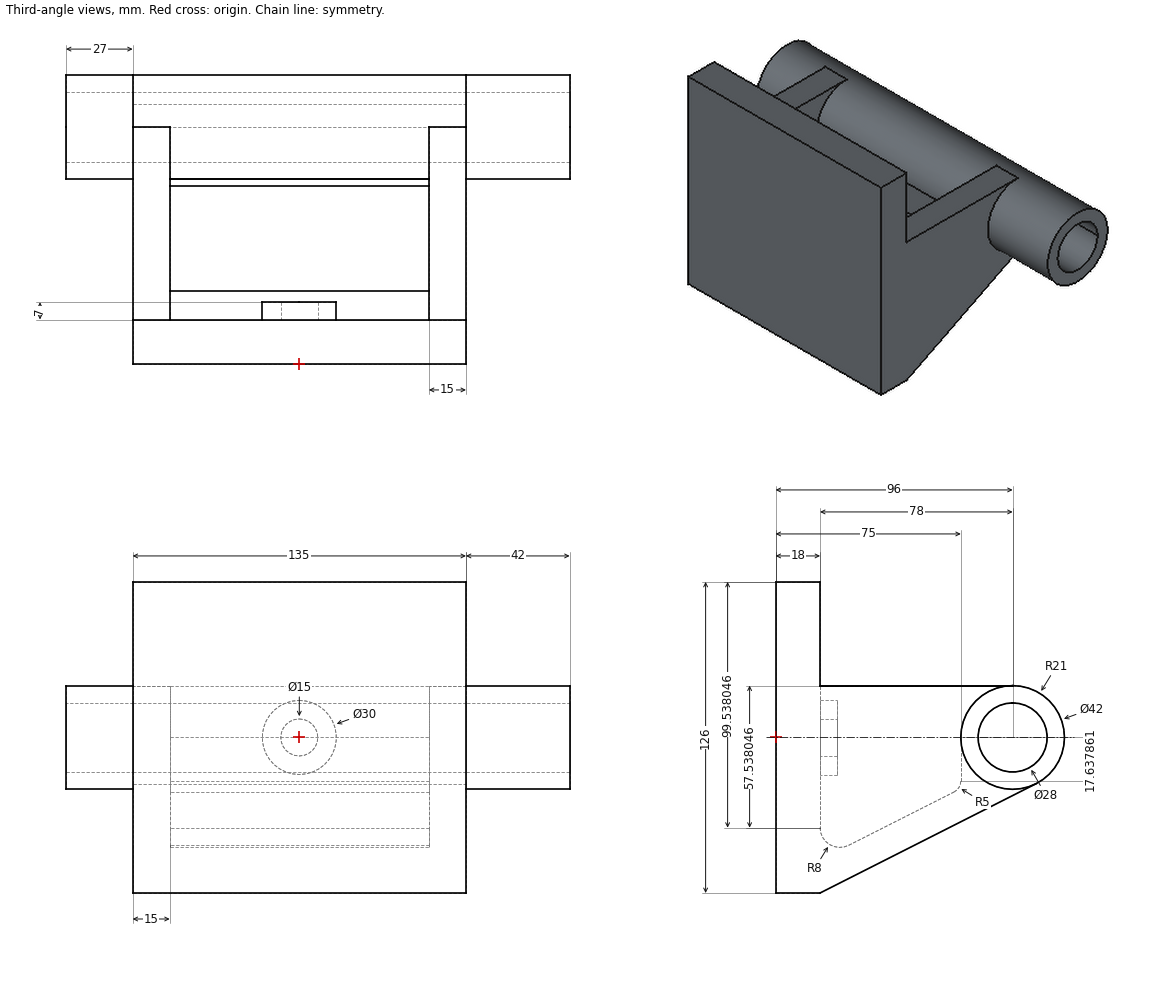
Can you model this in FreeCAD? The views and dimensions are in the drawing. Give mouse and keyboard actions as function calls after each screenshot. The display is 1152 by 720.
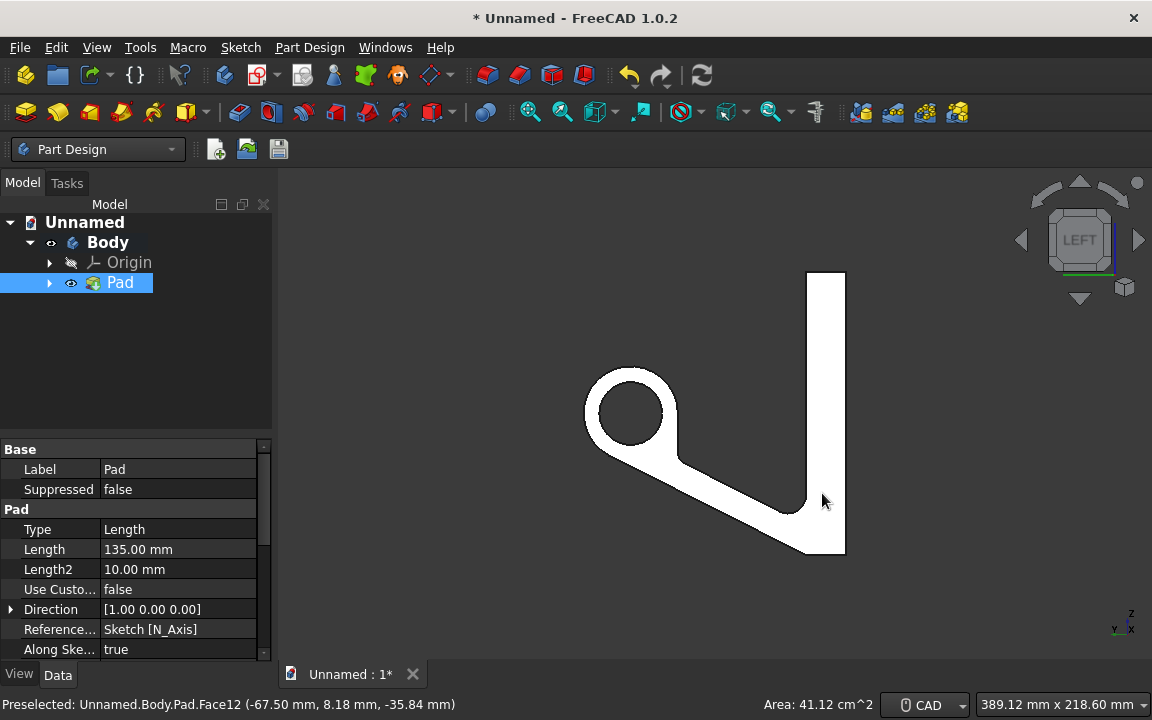
click(258, 76)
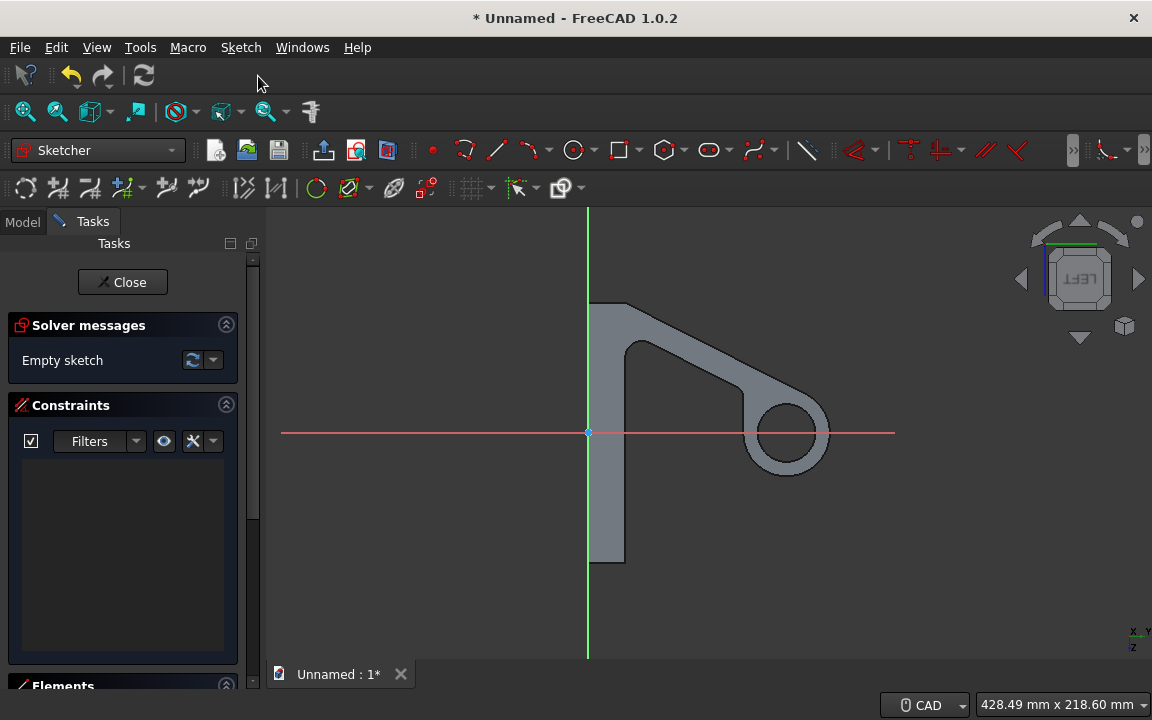
scroll(850, 433, up, 6)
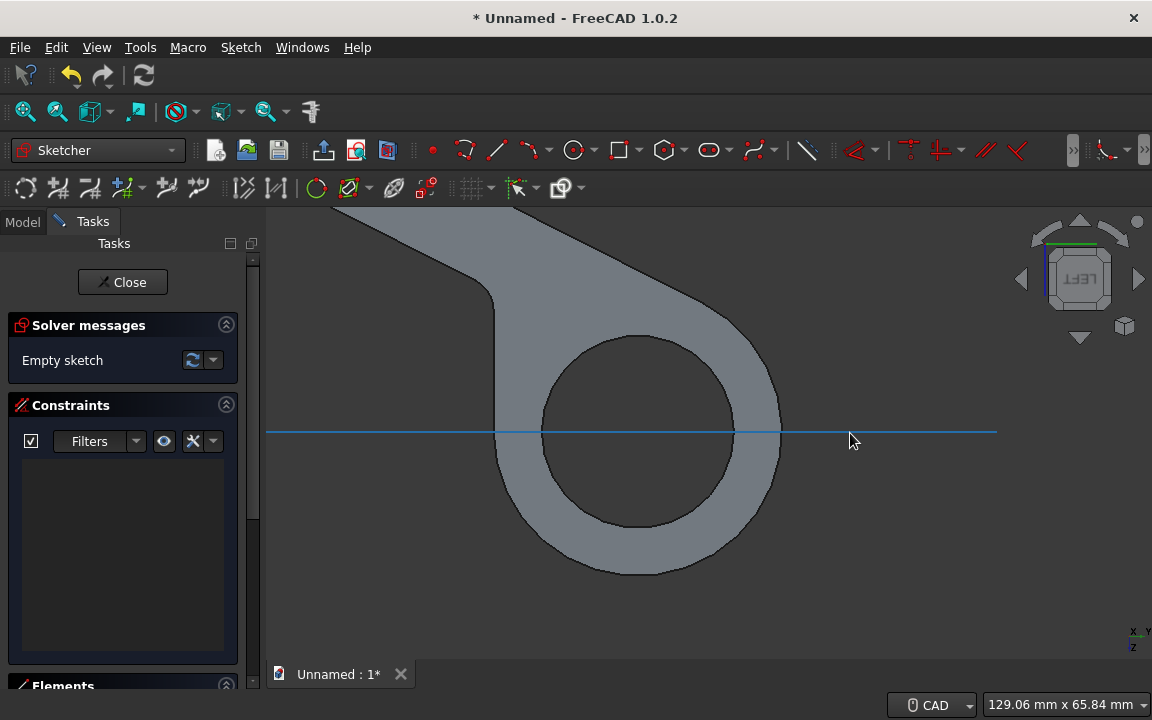
click(574, 150)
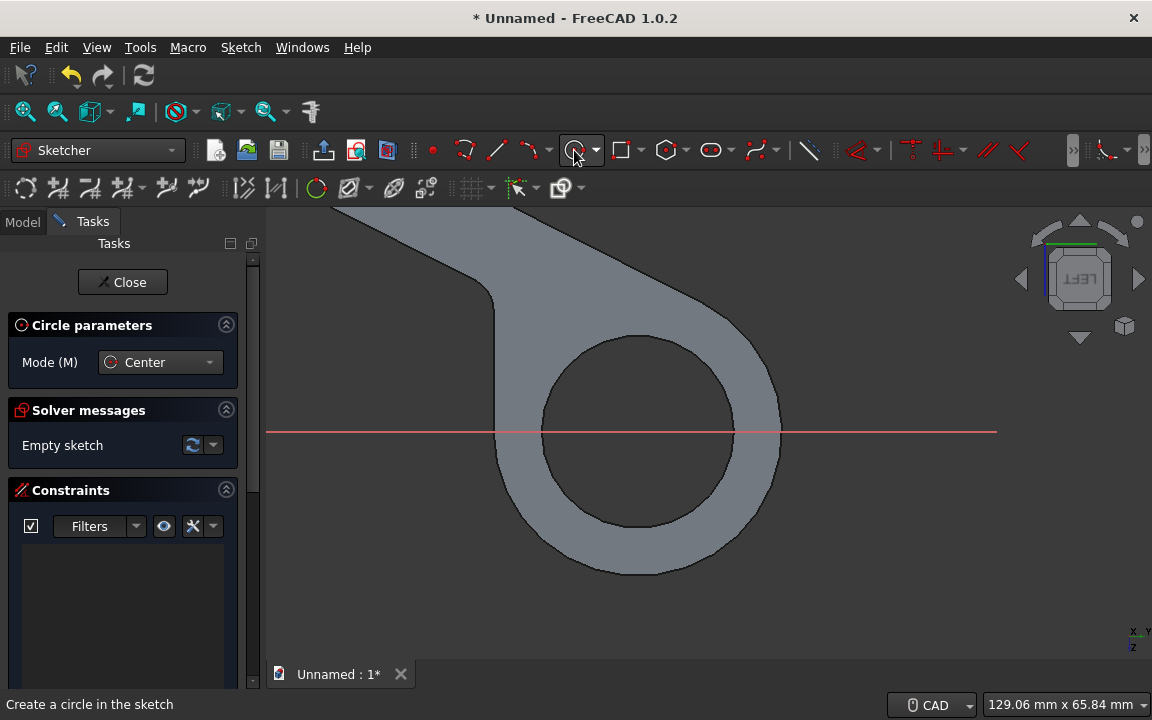
click(638, 432)
click(740, 330)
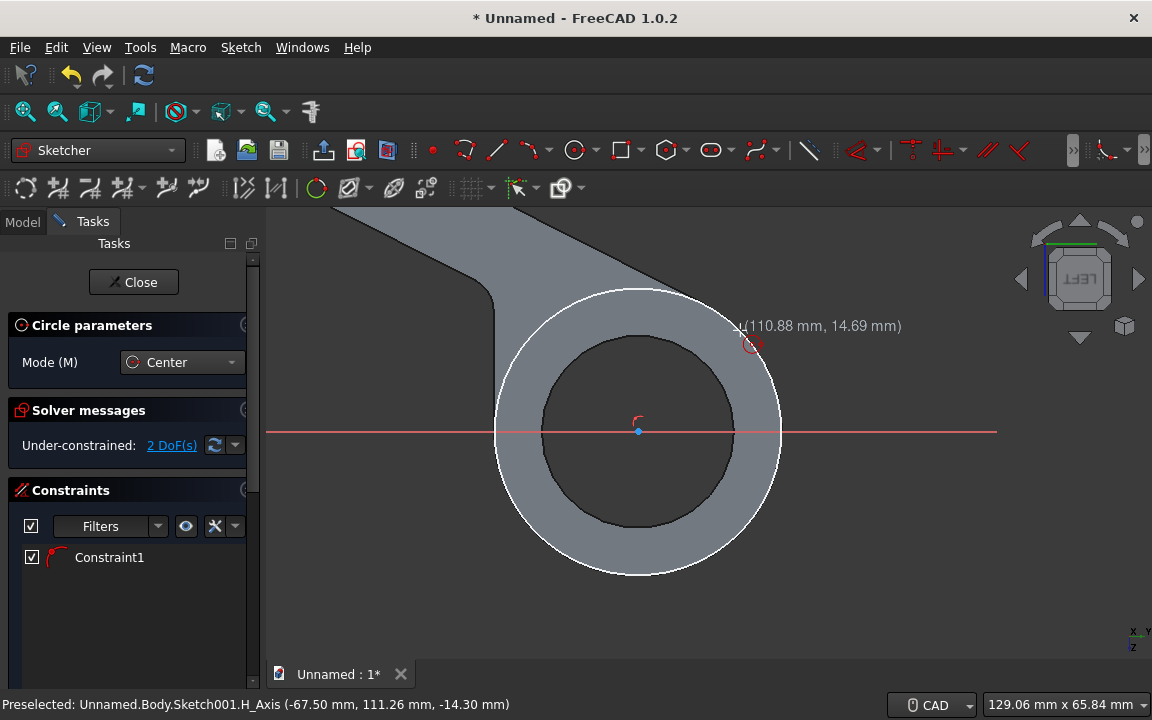
click(638, 432)
click(706, 364)
key(Escape)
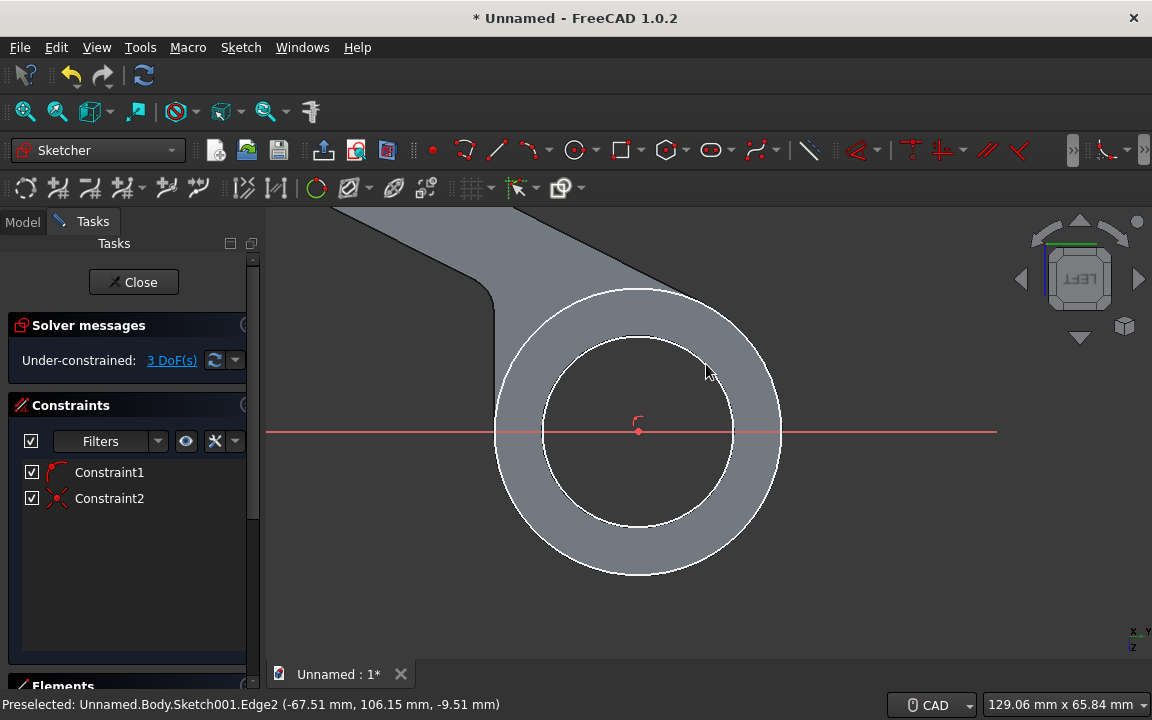
click(856, 150)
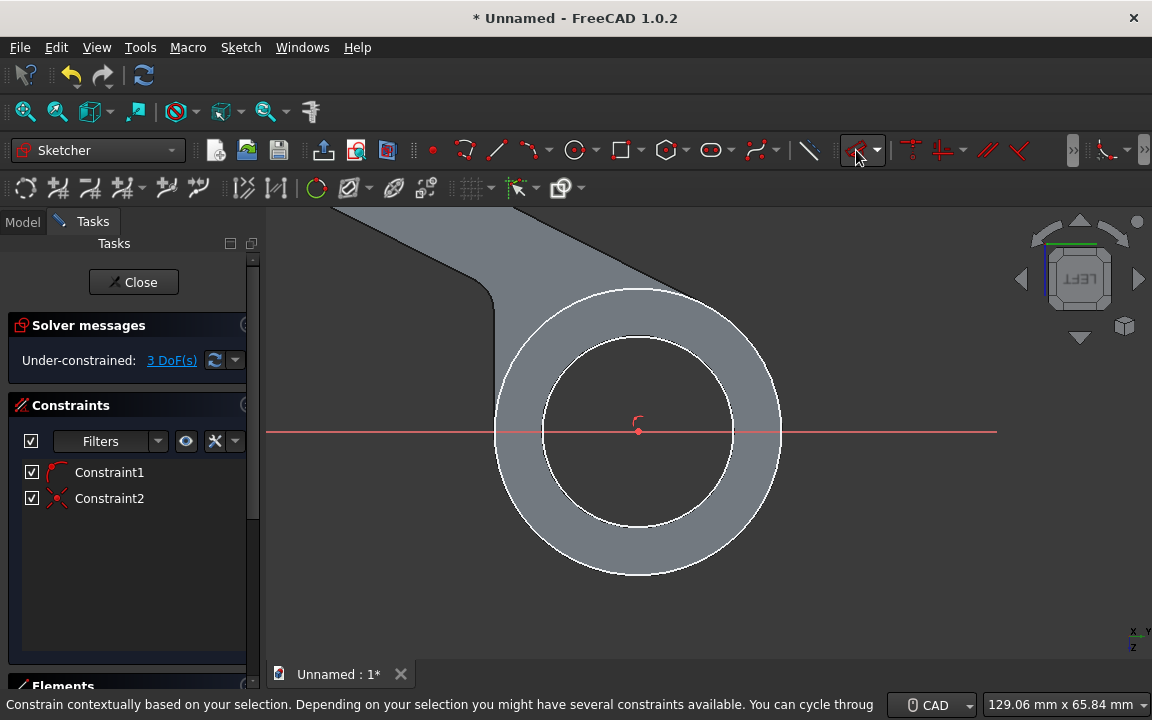
click(739, 330)
click(762, 307)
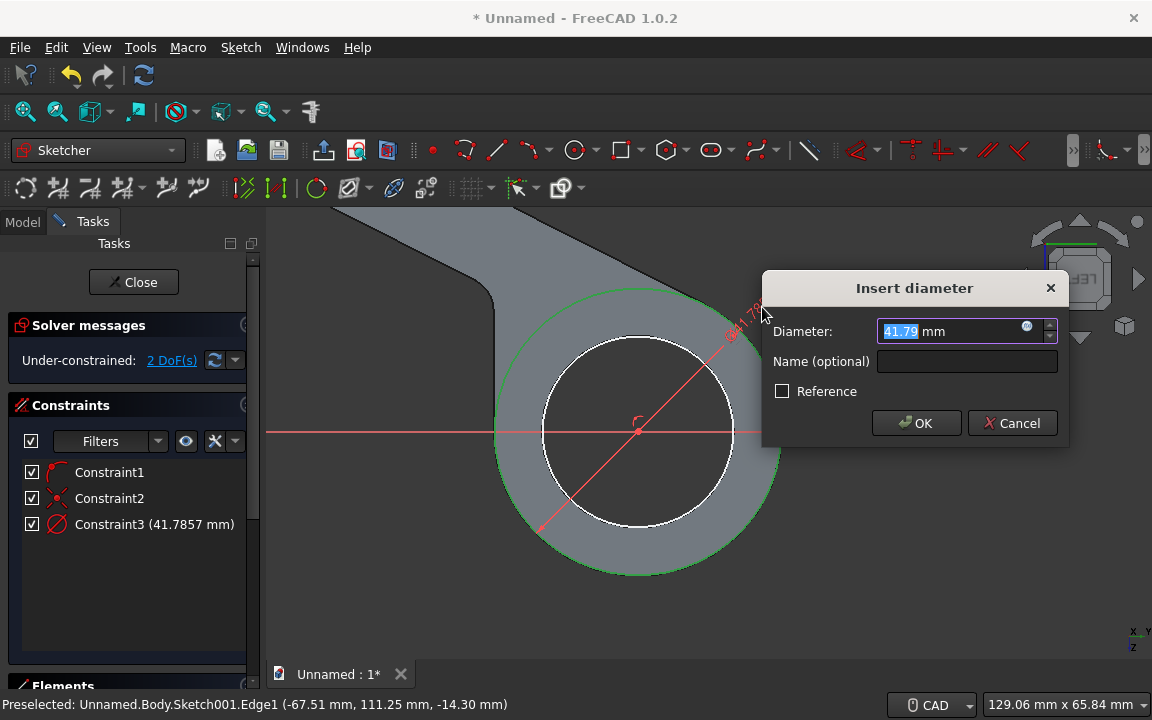
text(42)
key(Return)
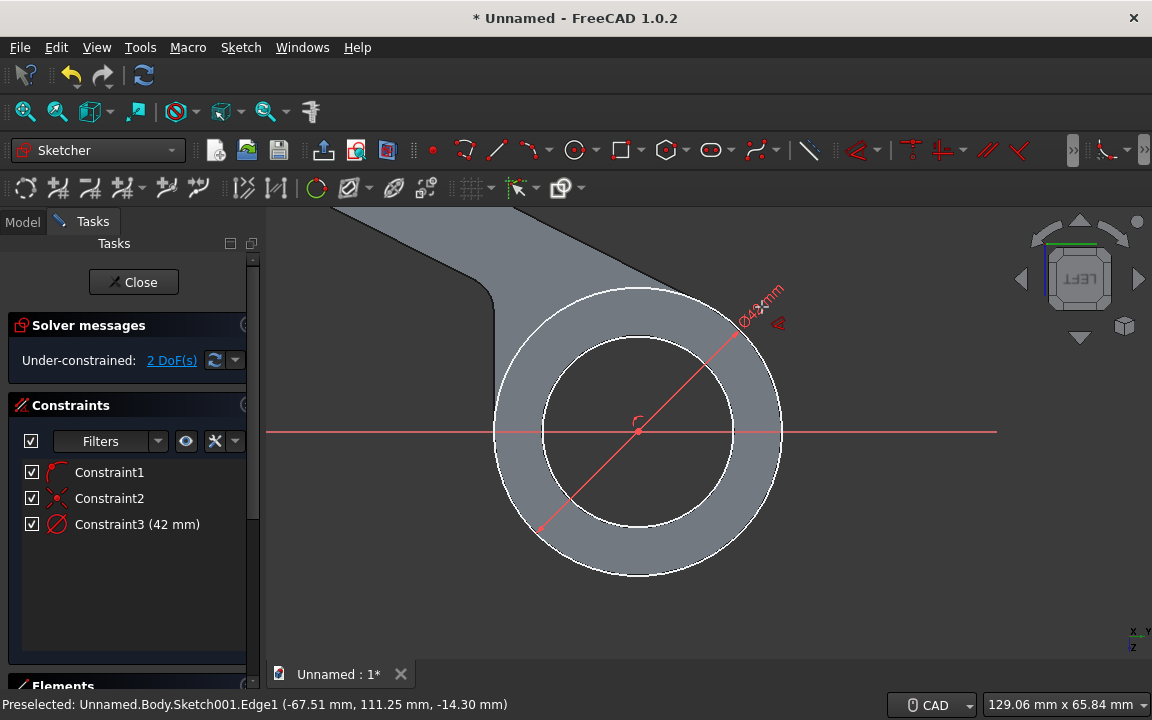
click(705, 364)
click(727, 341)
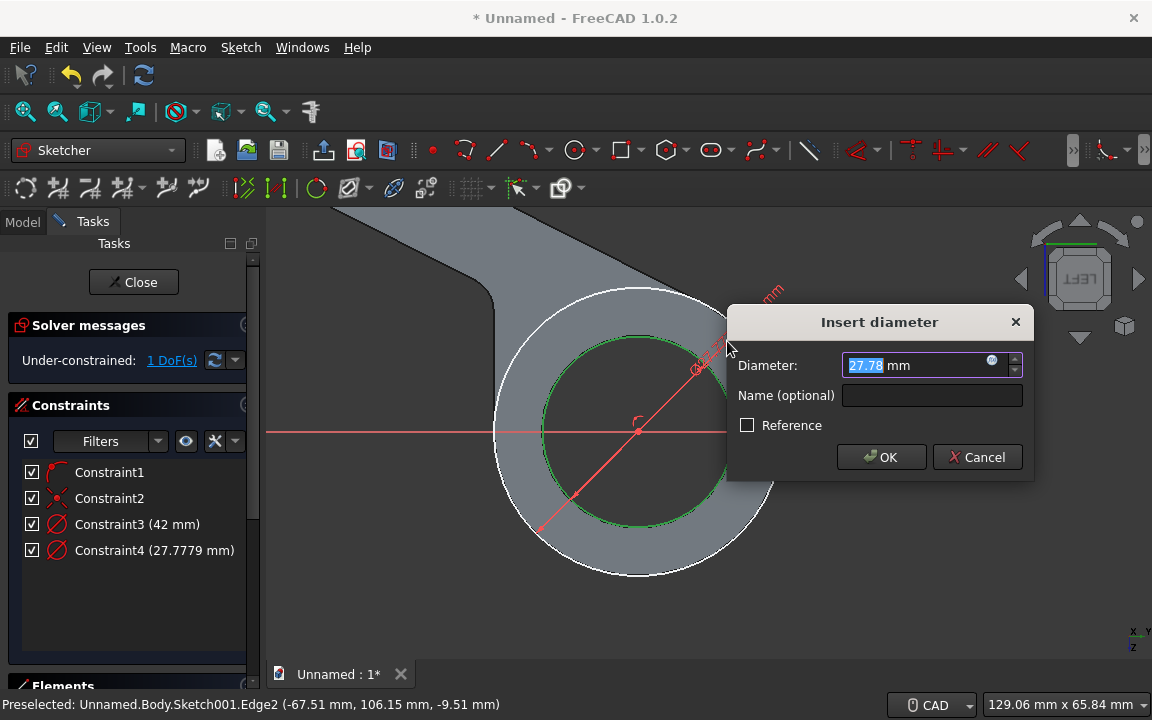
text(28)
key(Return)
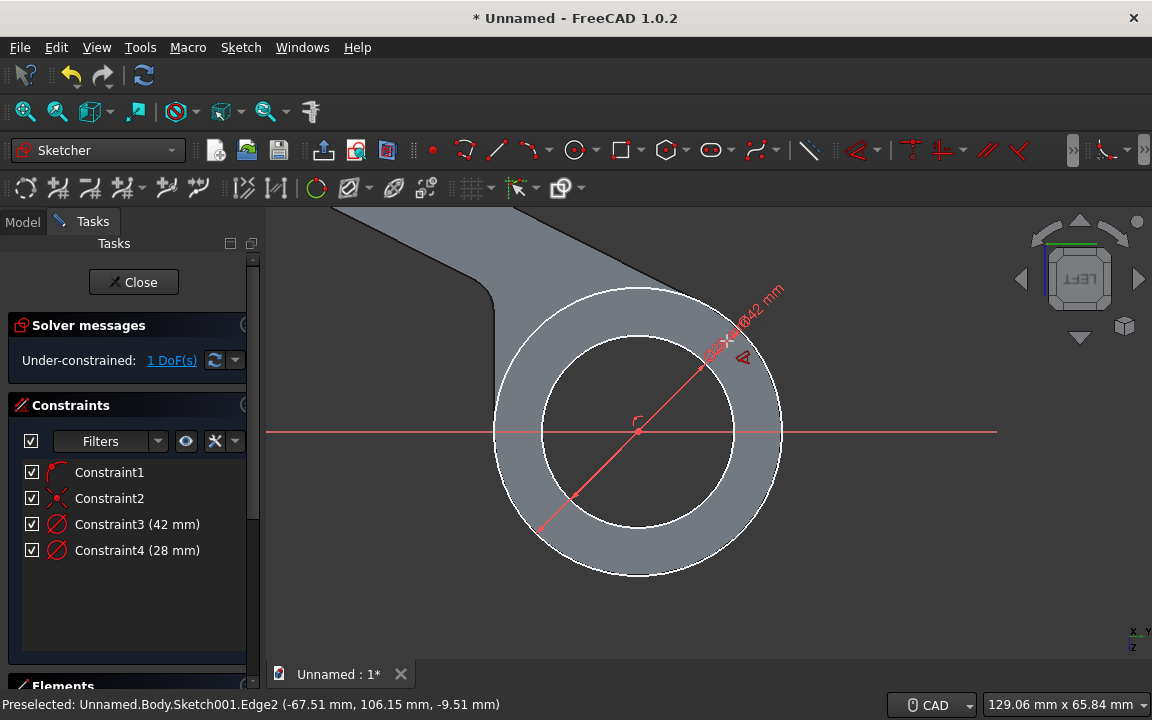
click(638, 432)
click(466, 466)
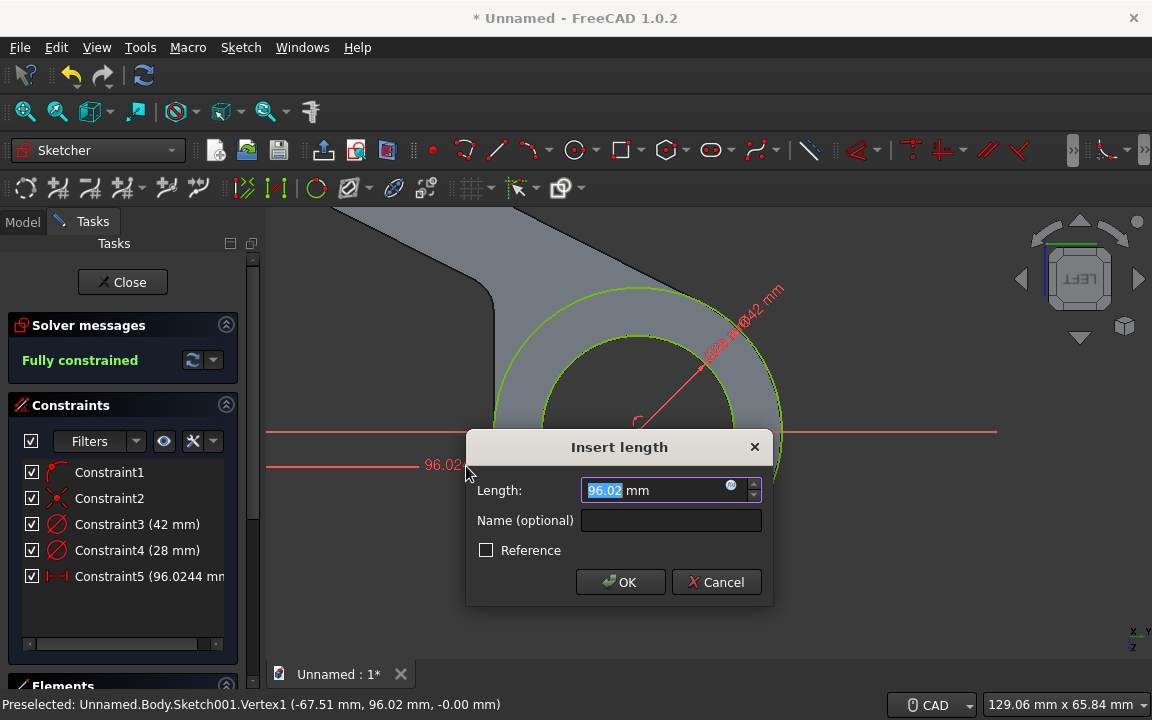
text(96)
key(Return)
key(Escape)